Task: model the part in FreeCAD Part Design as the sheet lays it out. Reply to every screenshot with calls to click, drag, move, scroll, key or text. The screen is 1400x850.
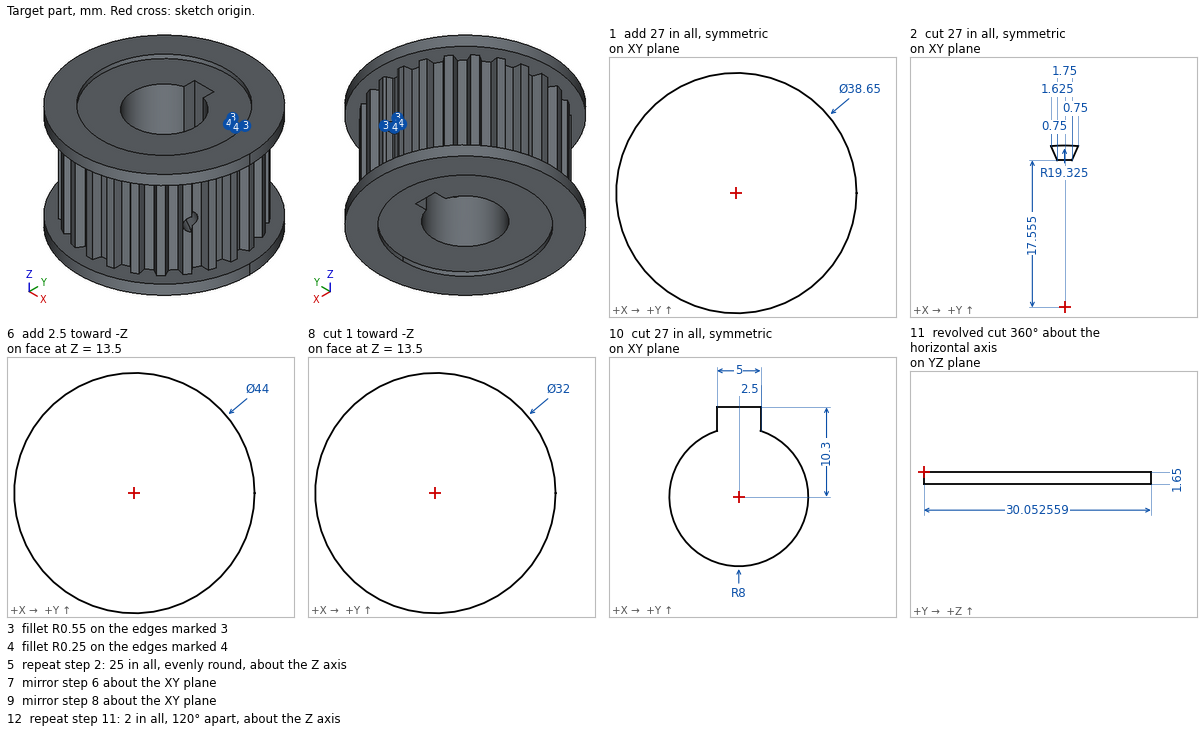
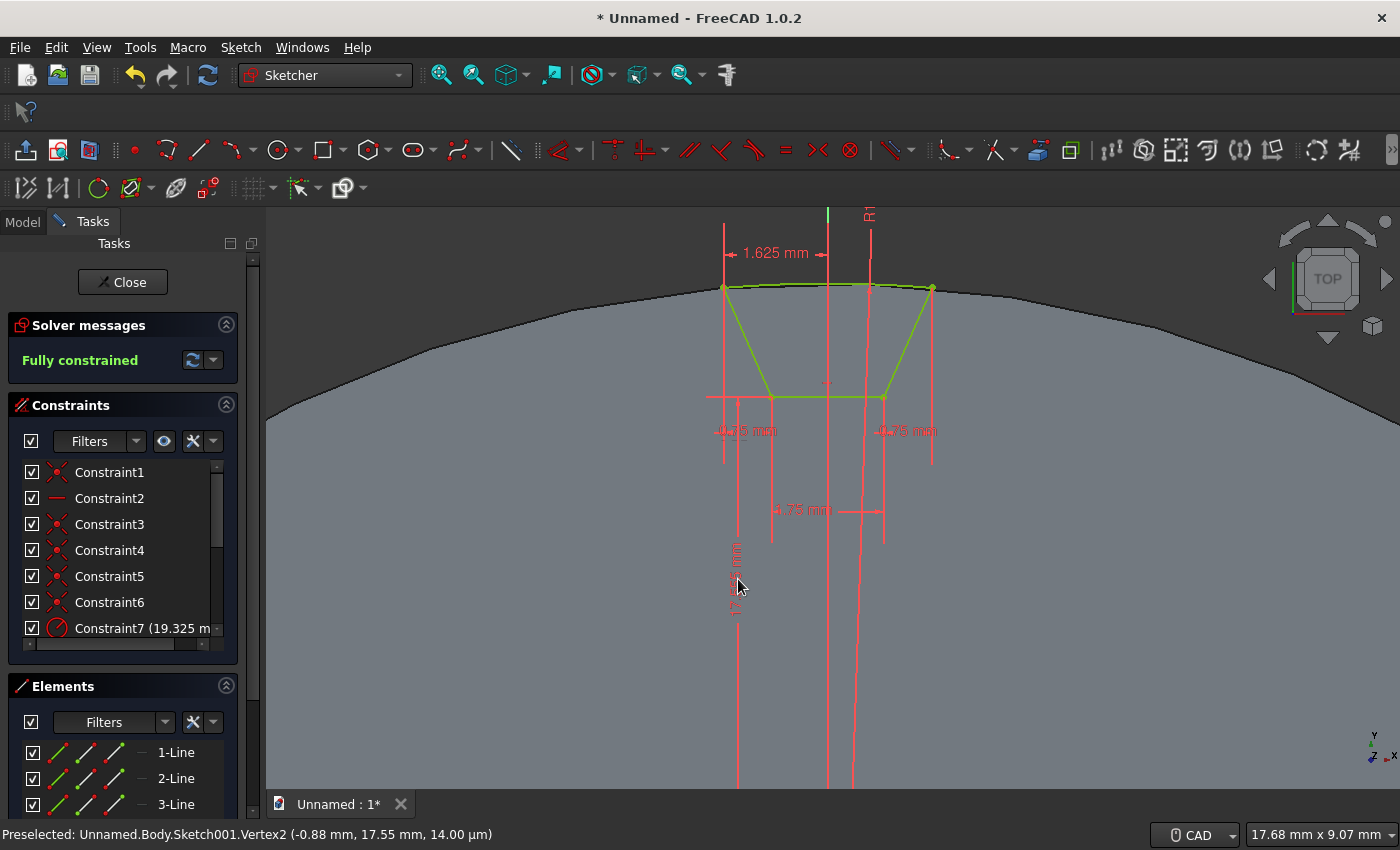
click(123, 282)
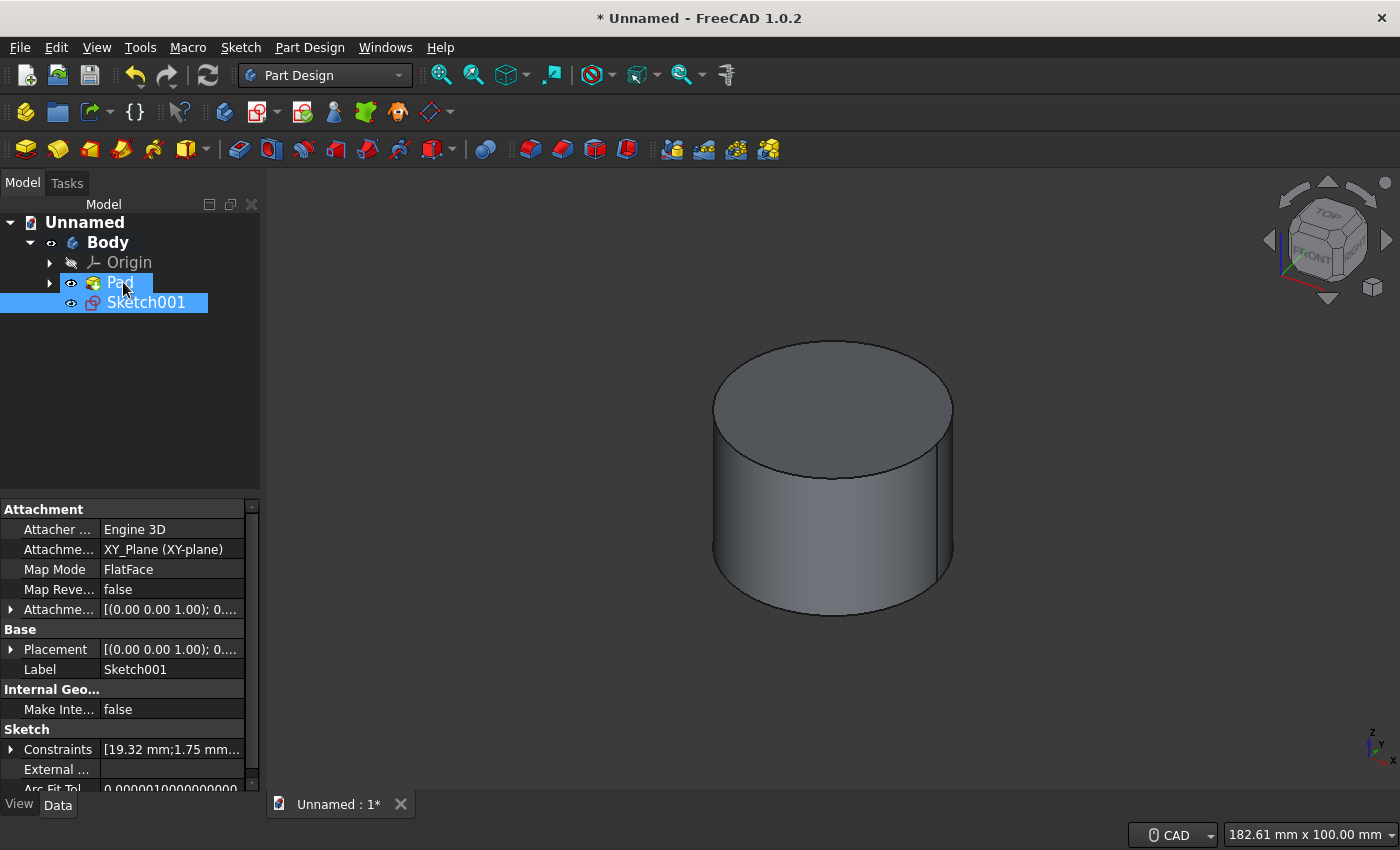
click(240, 150)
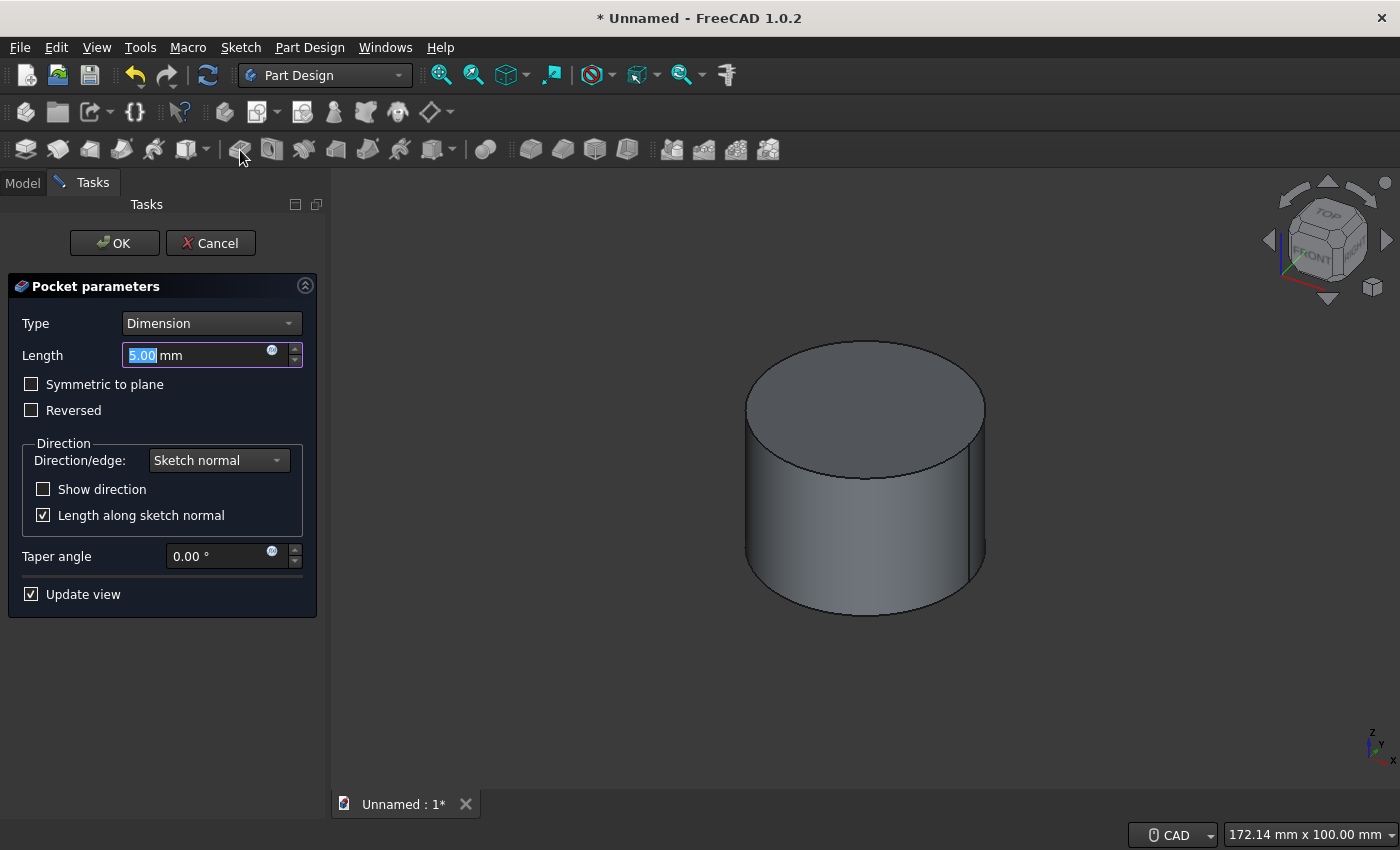
text(27)
key(Tab)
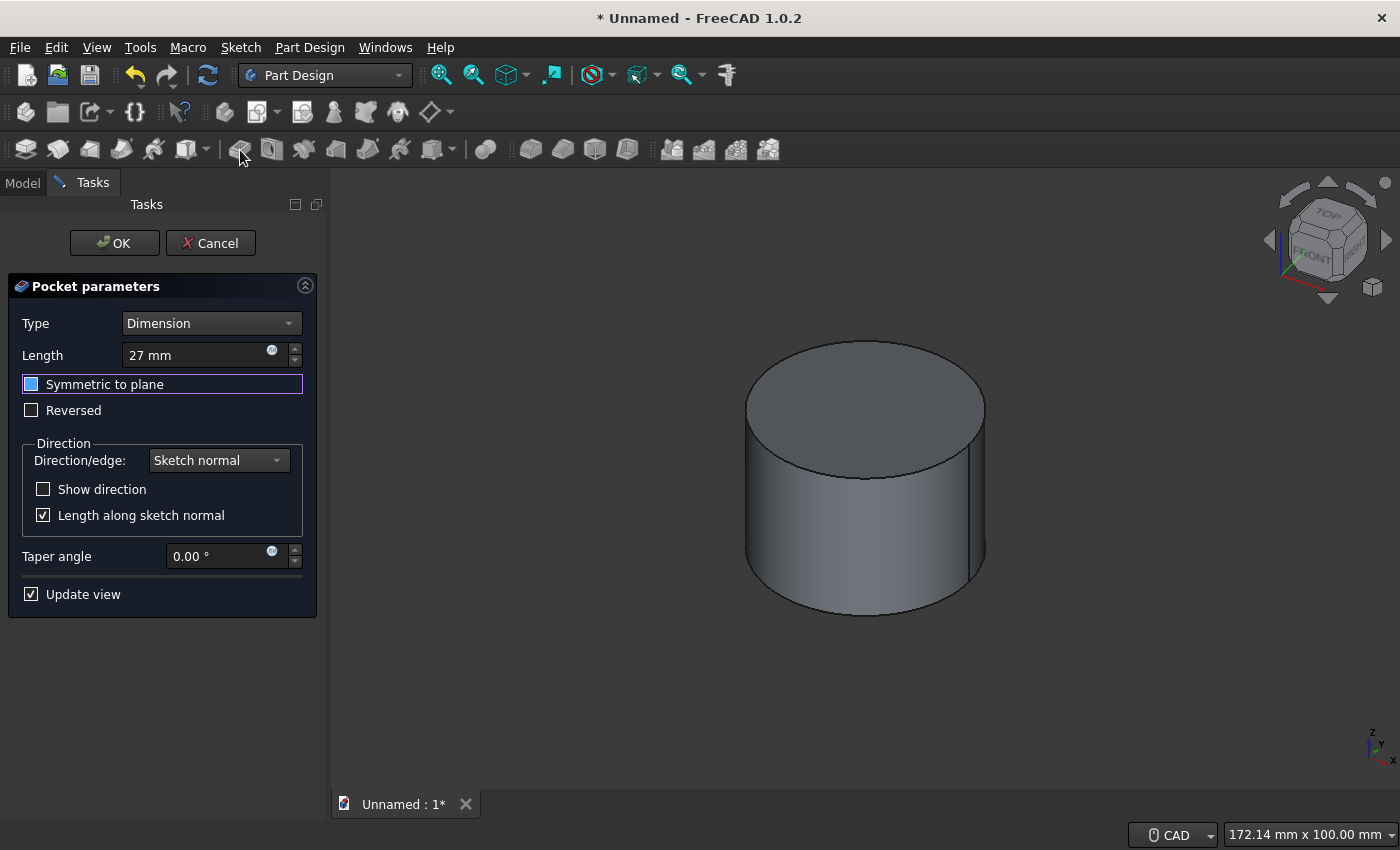
click(30, 384)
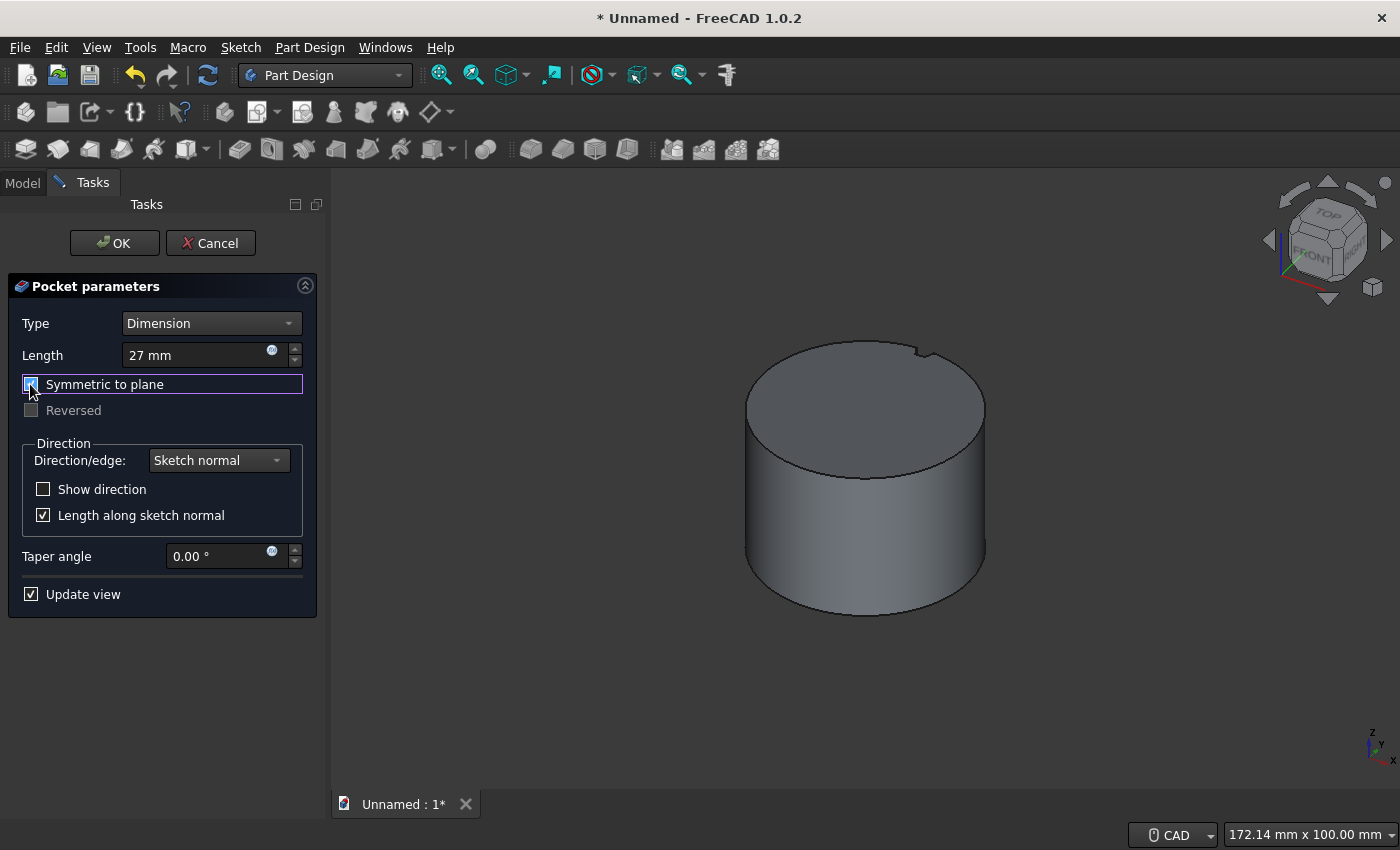
click(115, 243)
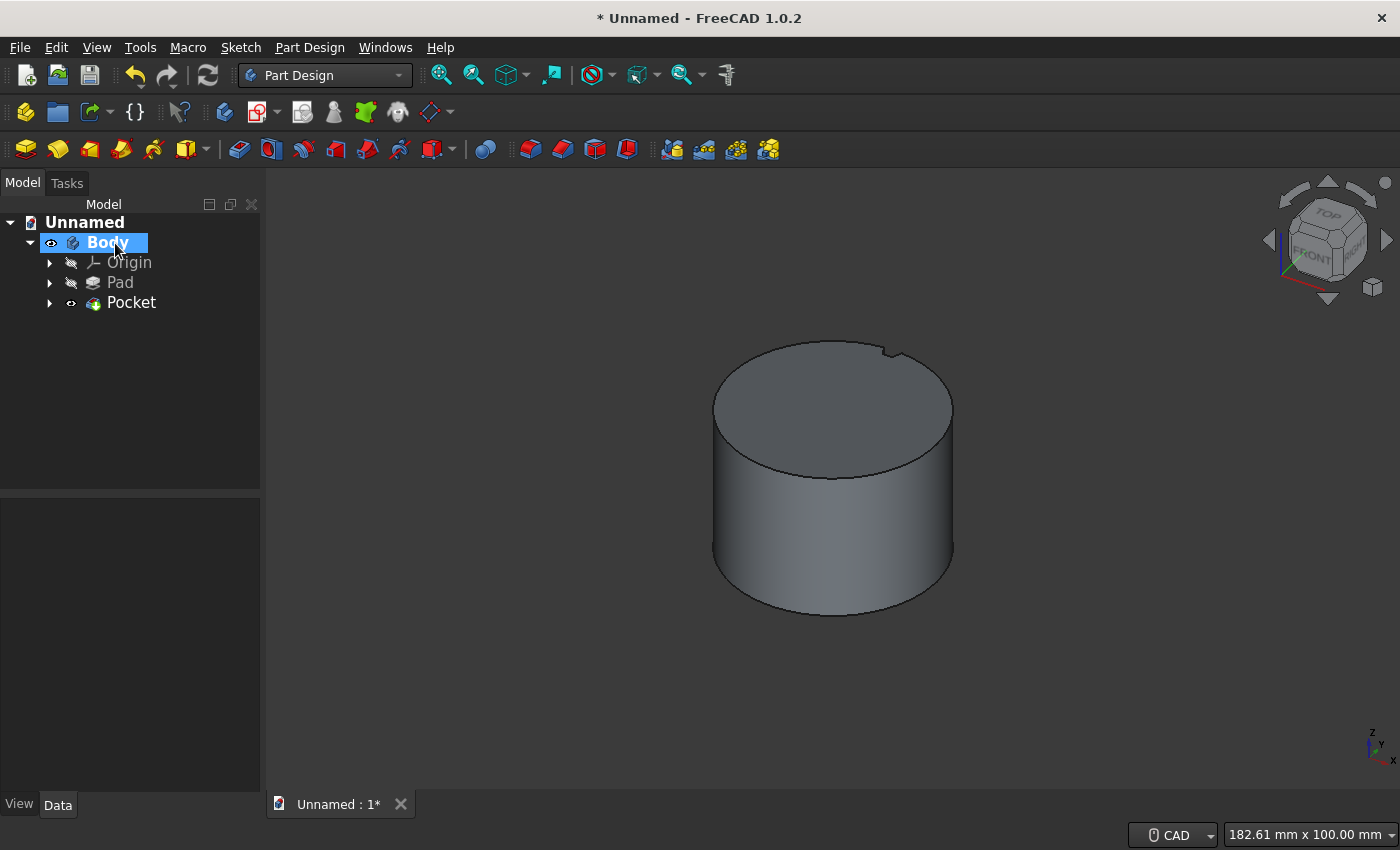
key(0)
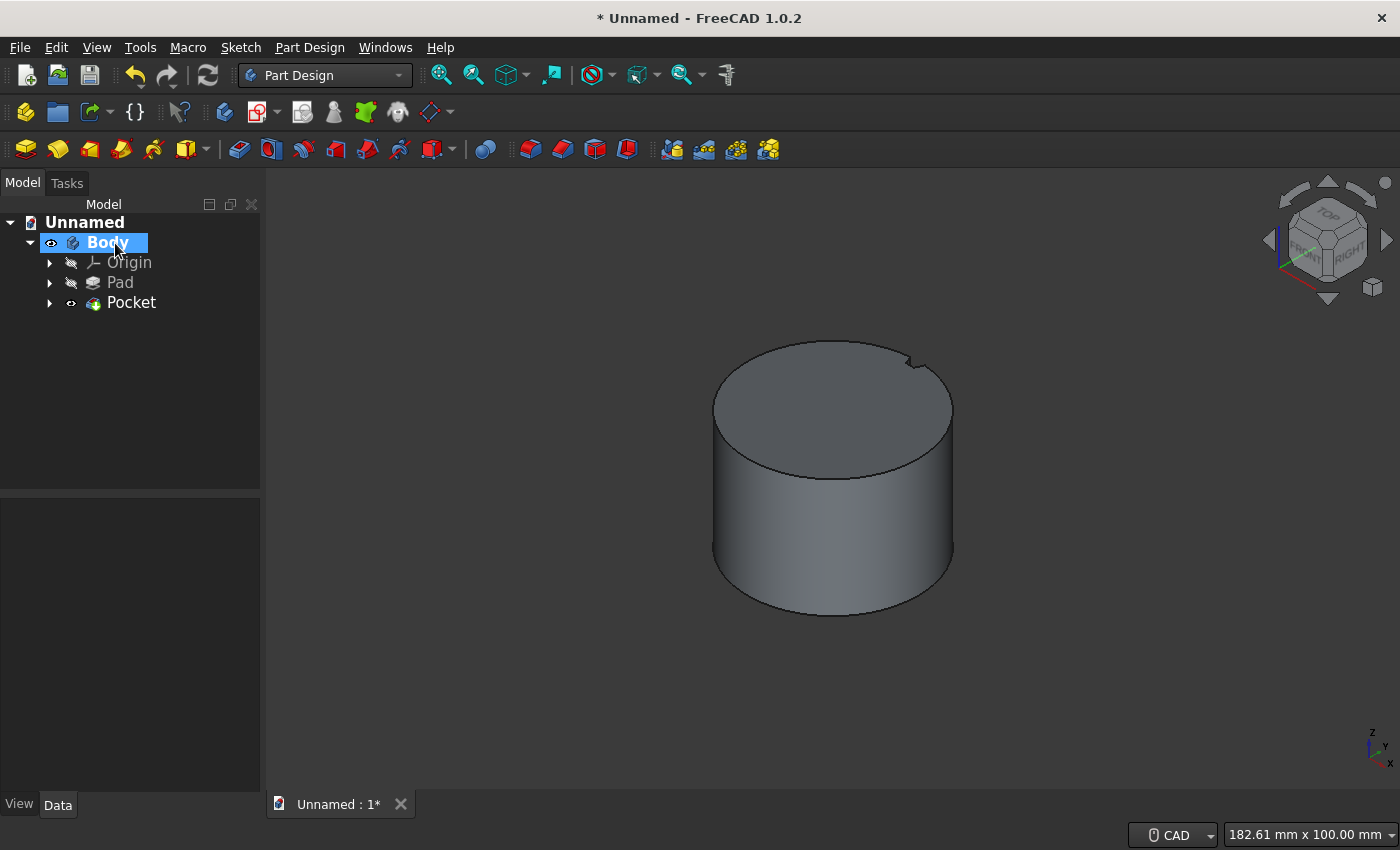
key(2)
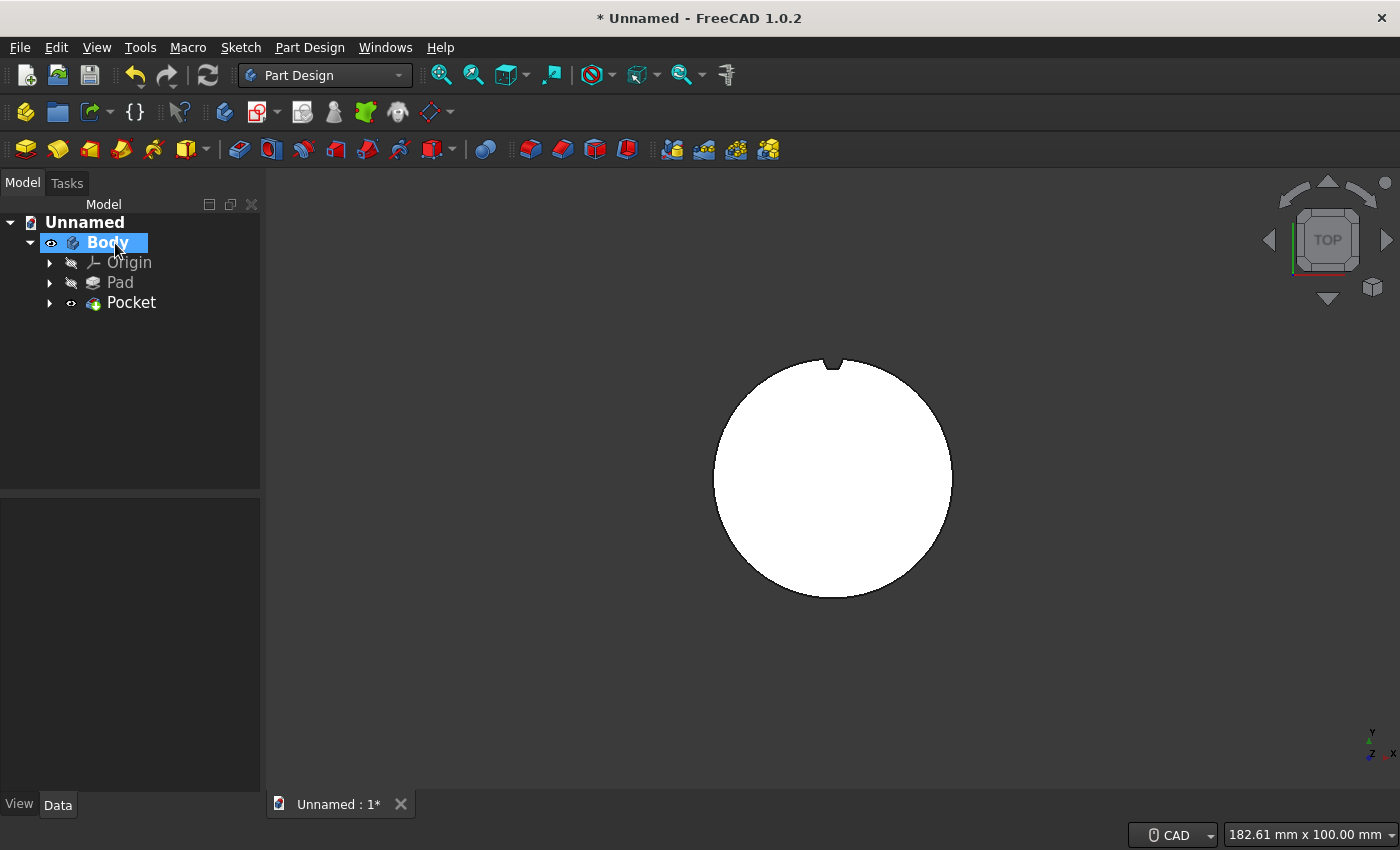
click(442, 76)